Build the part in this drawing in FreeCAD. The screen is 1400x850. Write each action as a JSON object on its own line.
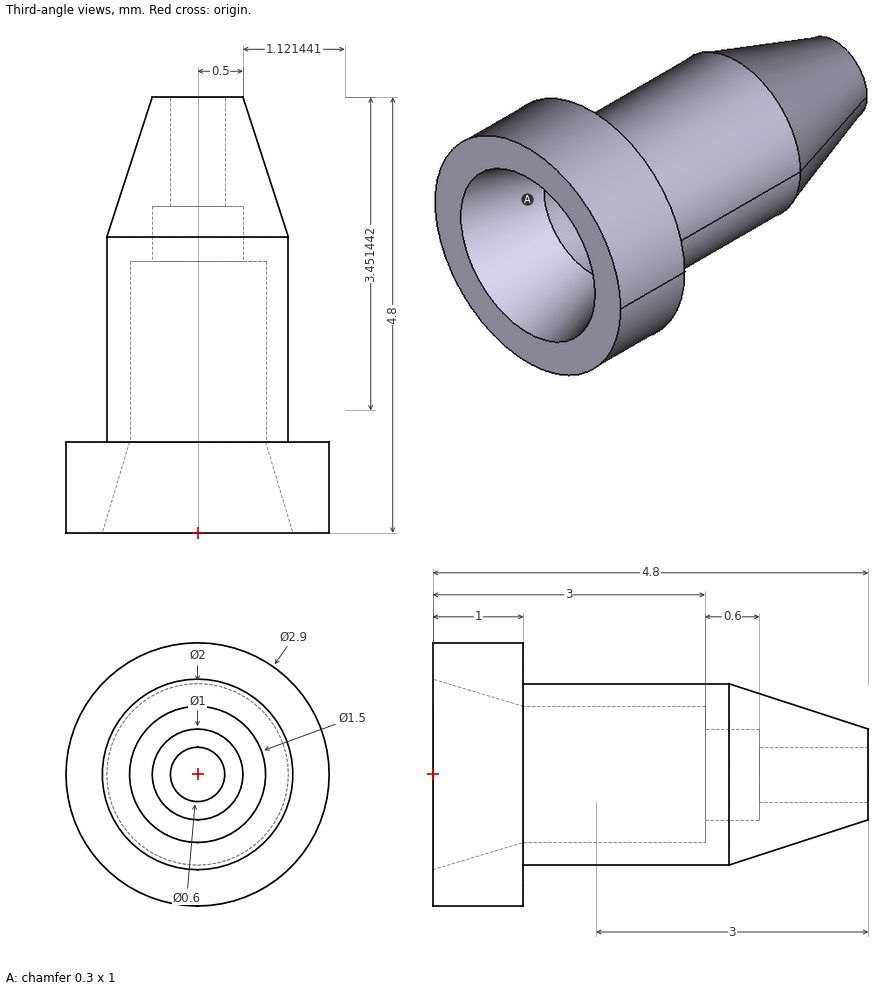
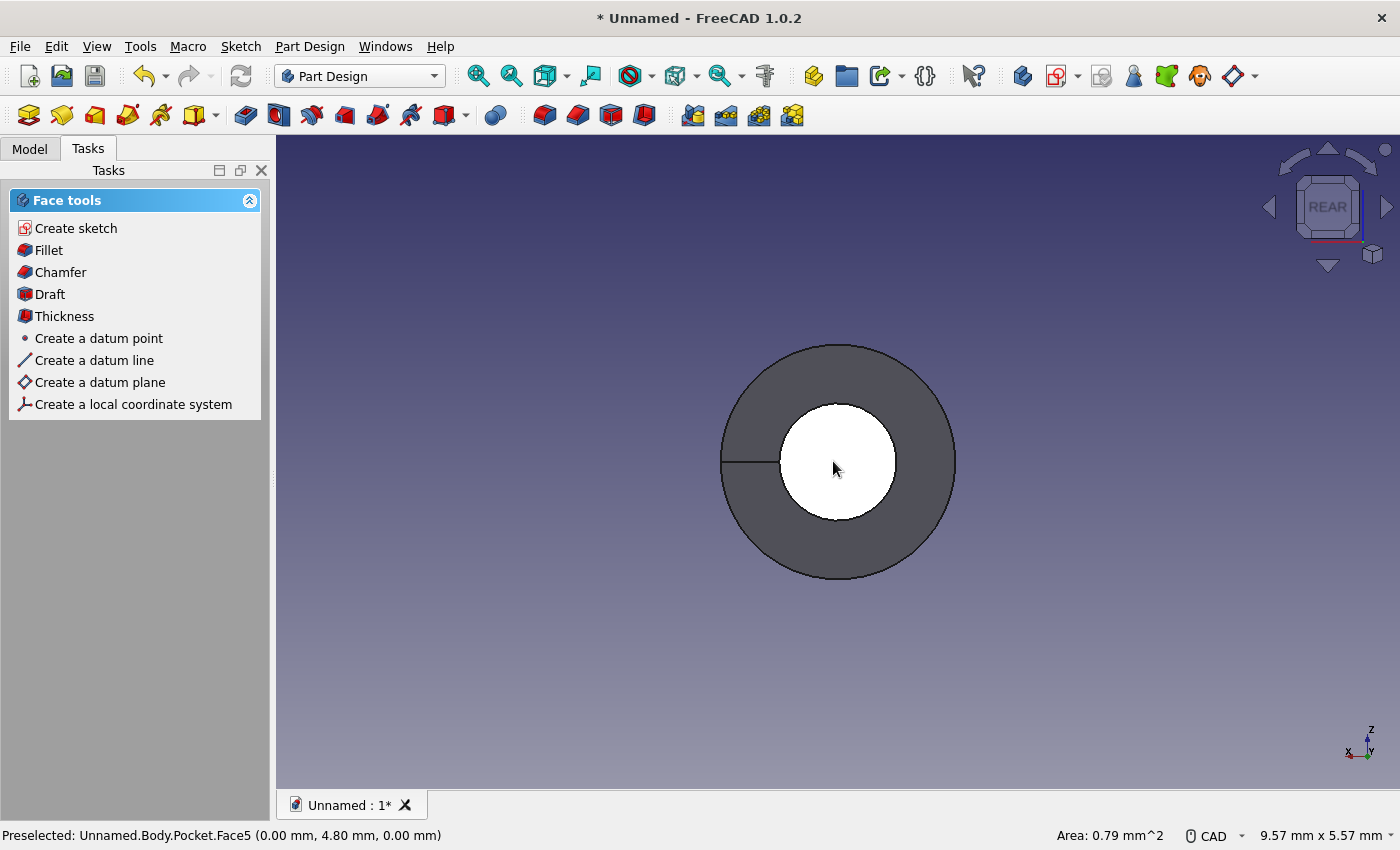
{"action": "left_click", "coordinate": [1056, 76]}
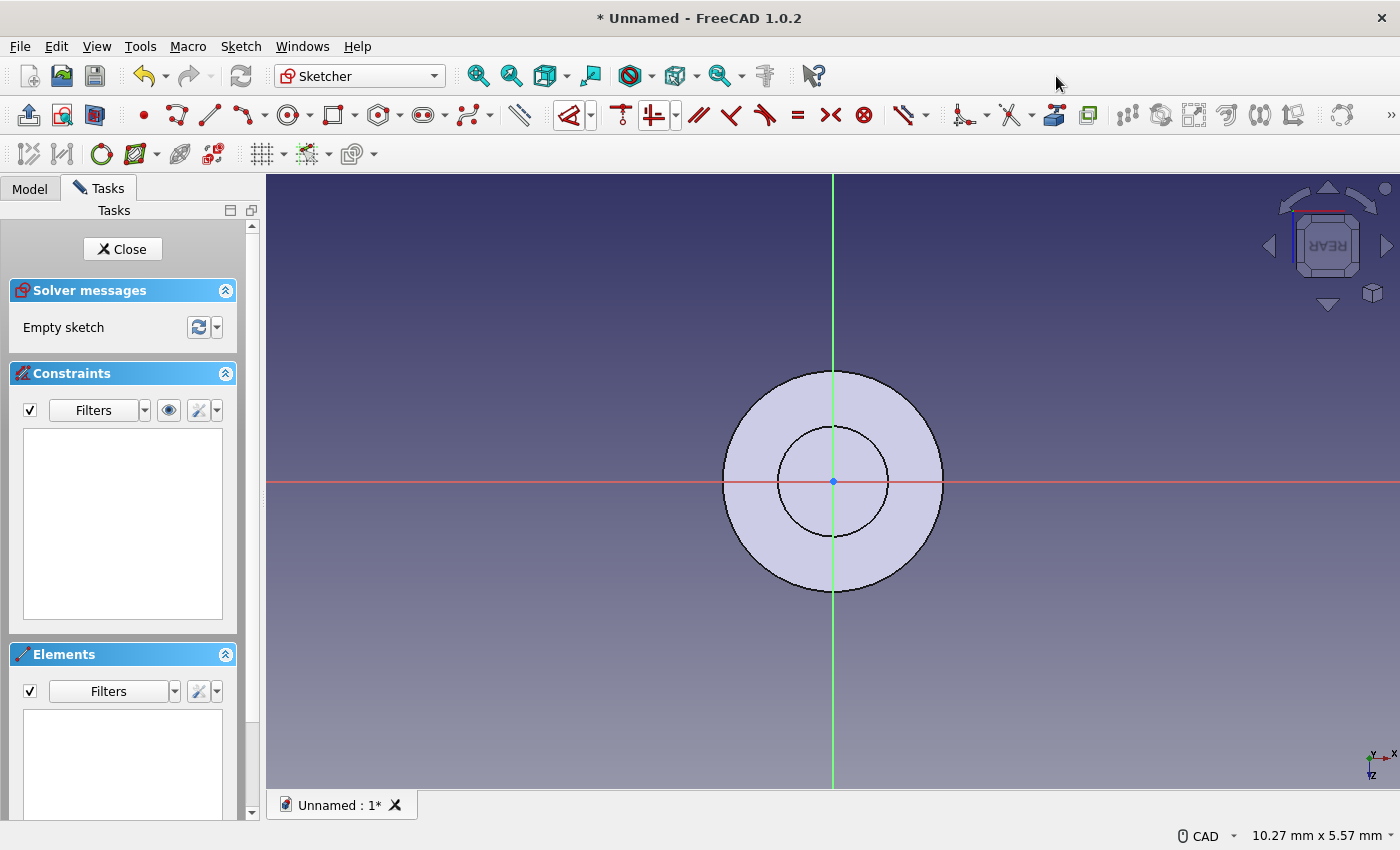
{"action": "scroll", "coordinate": [847, 481], "scroll_direction": "up", "scroll_amount": 9}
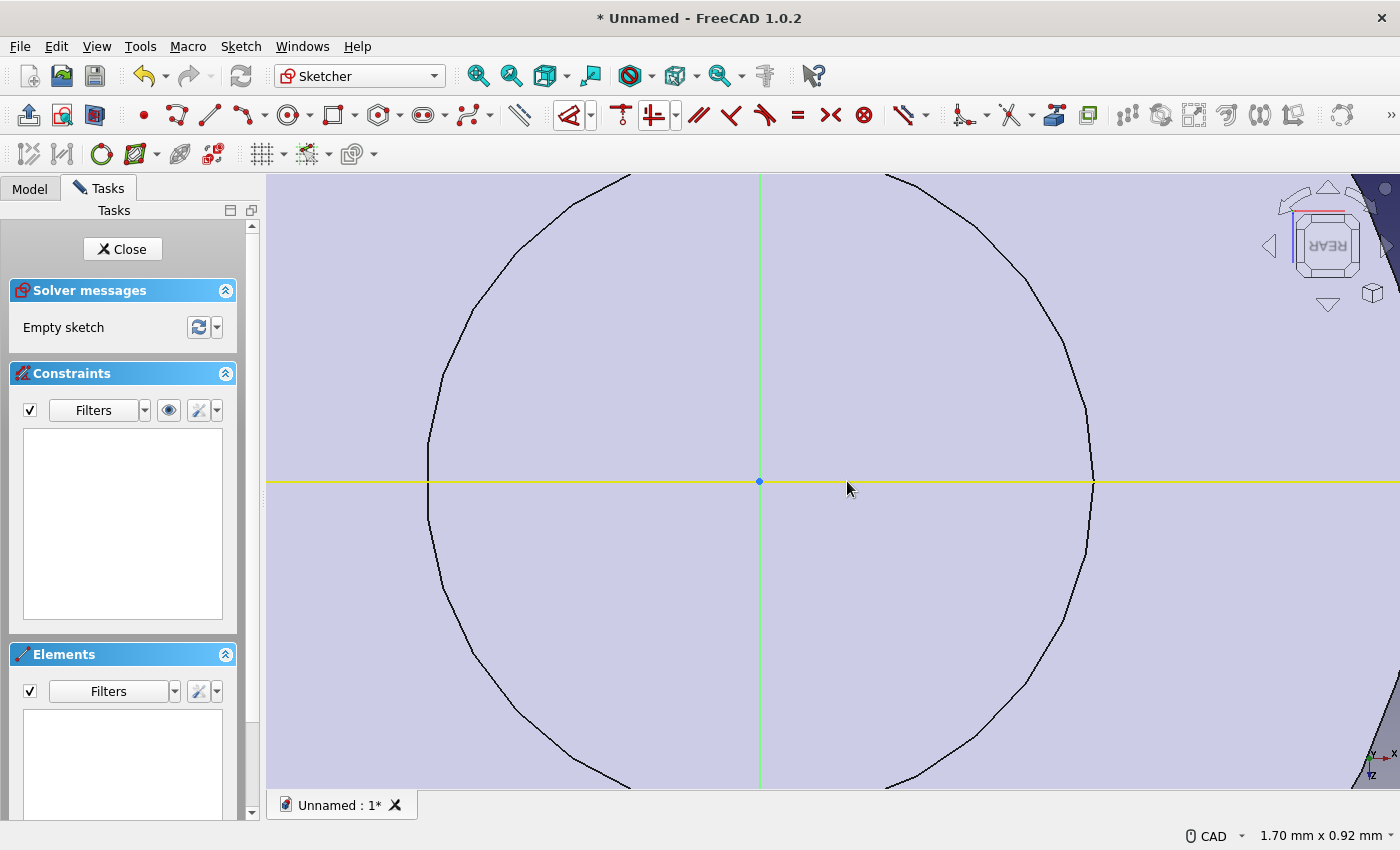
{"action": "left_click", "coordinate": [288, 116]}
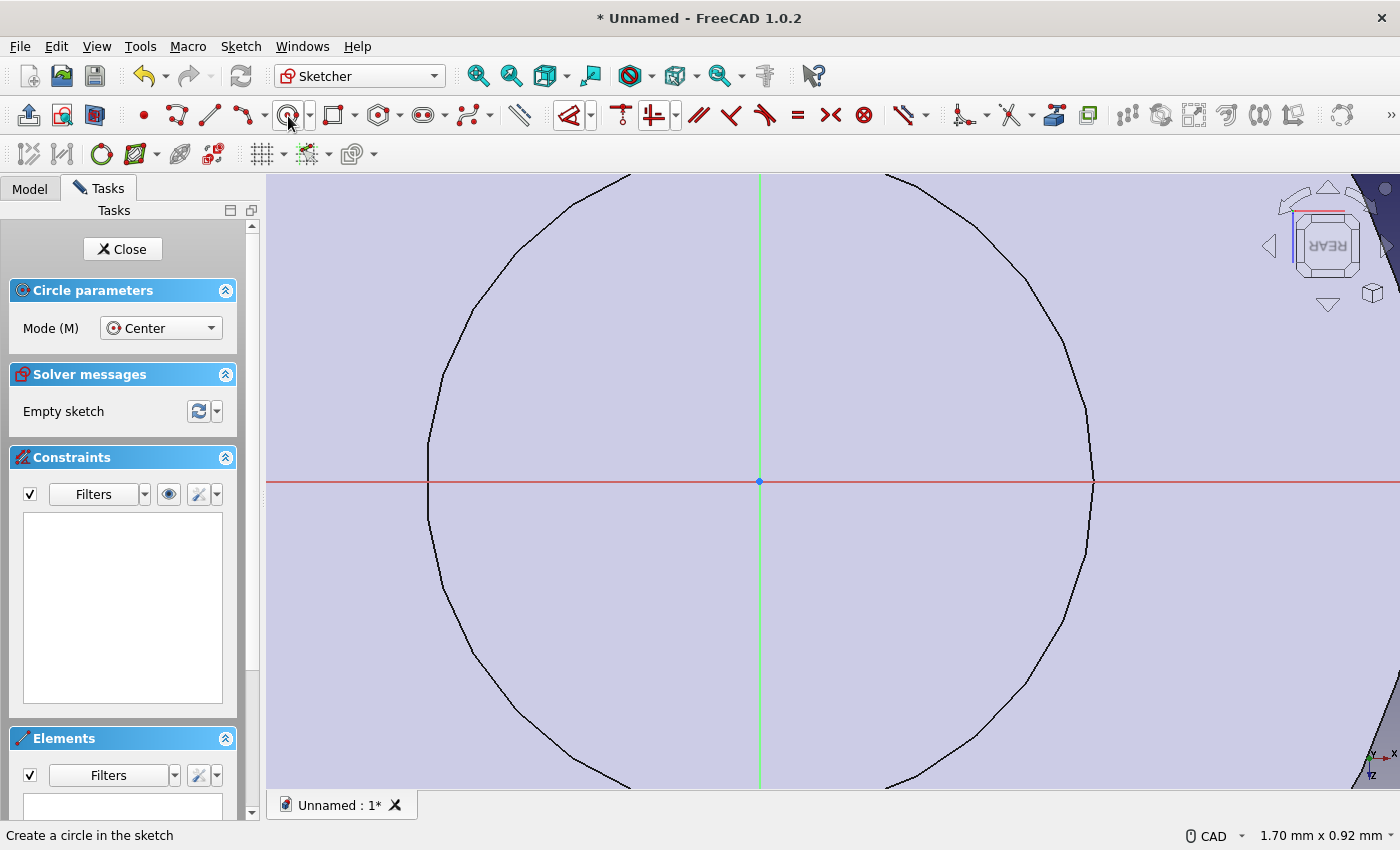
{"action": "left_click", "coordinate": [760, 481]}
{"action": "left_click", "coordinate": [901, 340]}
{"action": "key", "text": "Escape"}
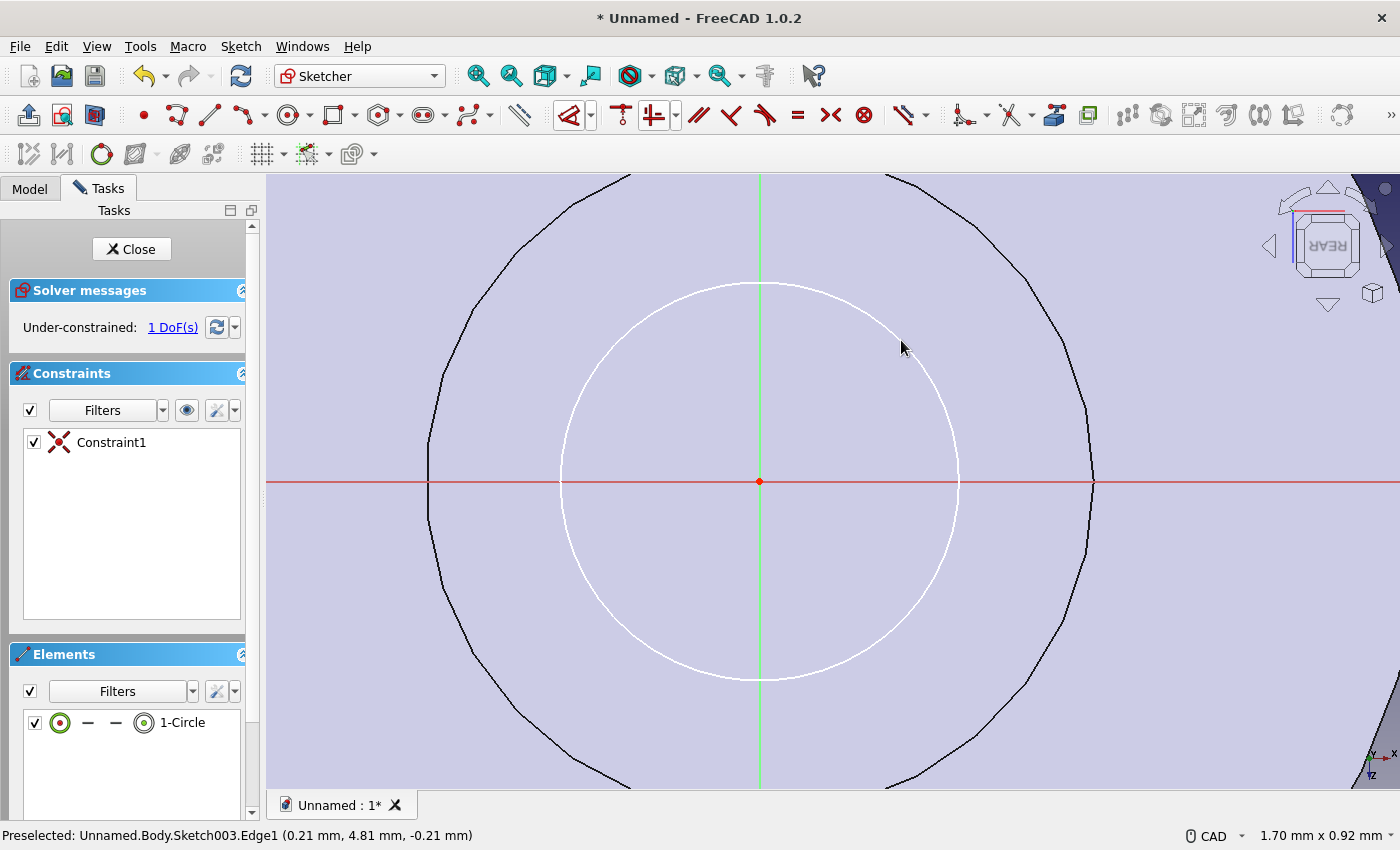
{"action": "left_click", "coordinate": [900, 340]}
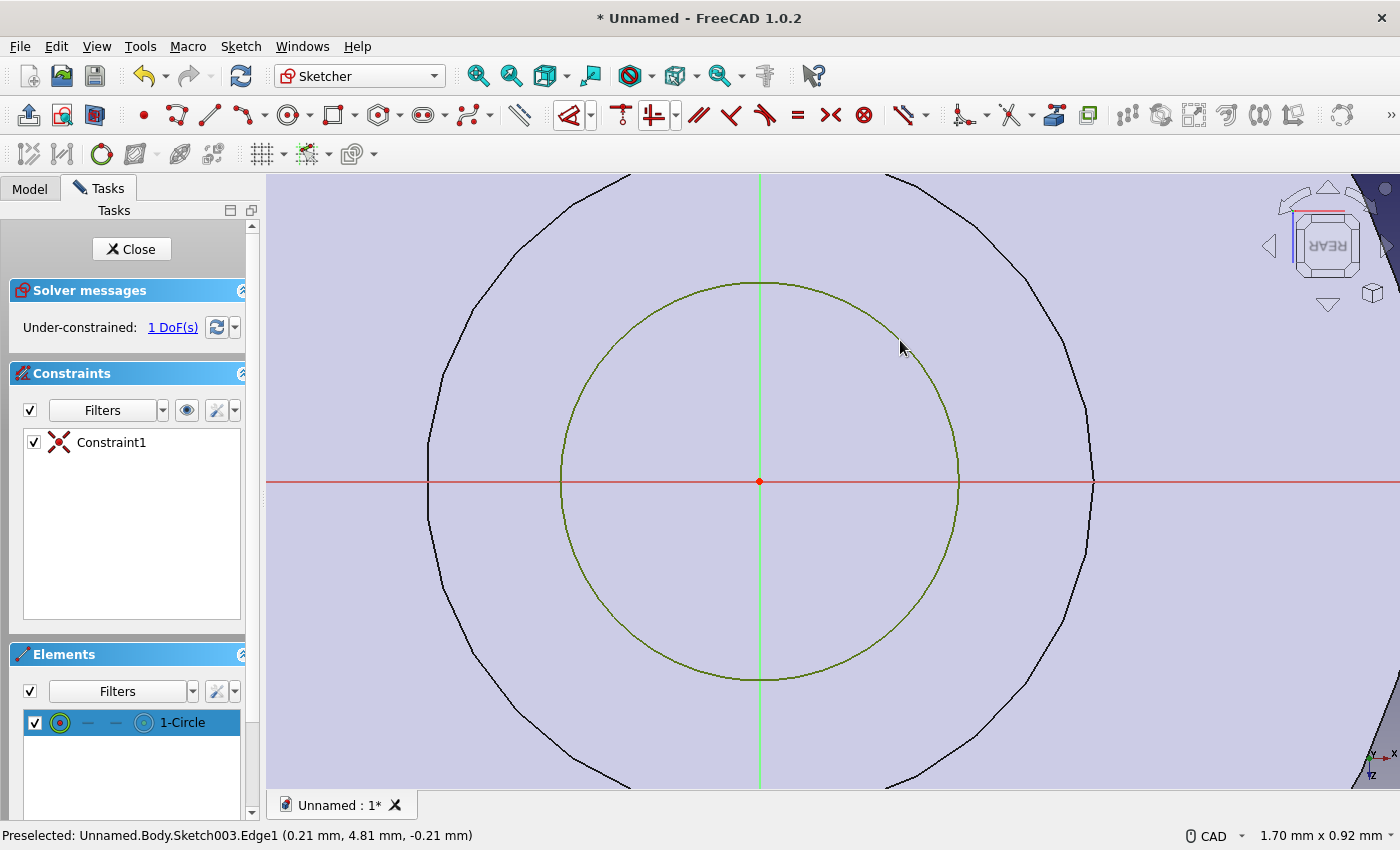
{"action": "left_click", "coordinate": [590, 116]}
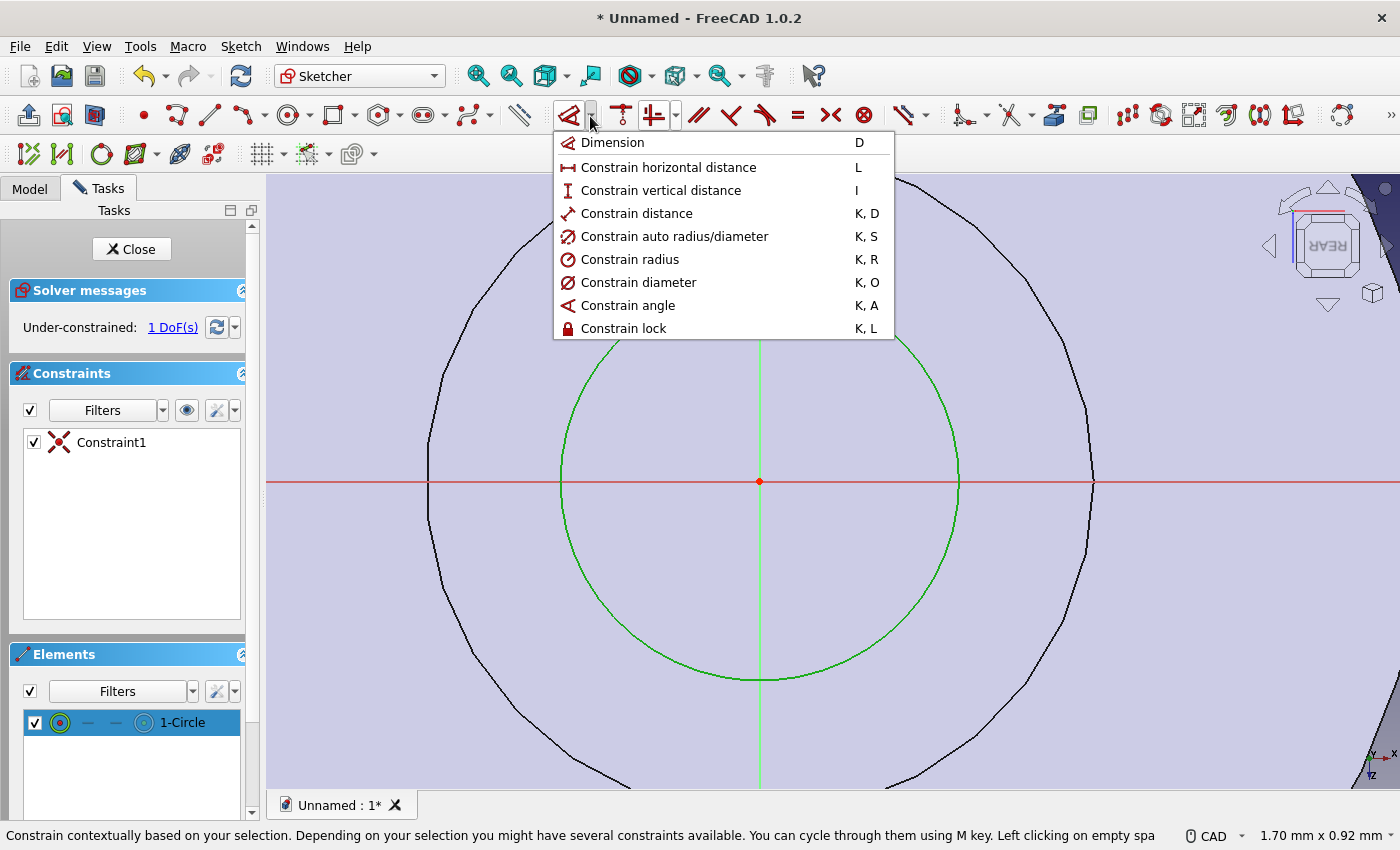
{"action": "left_click", "coordinate": [724, 282]}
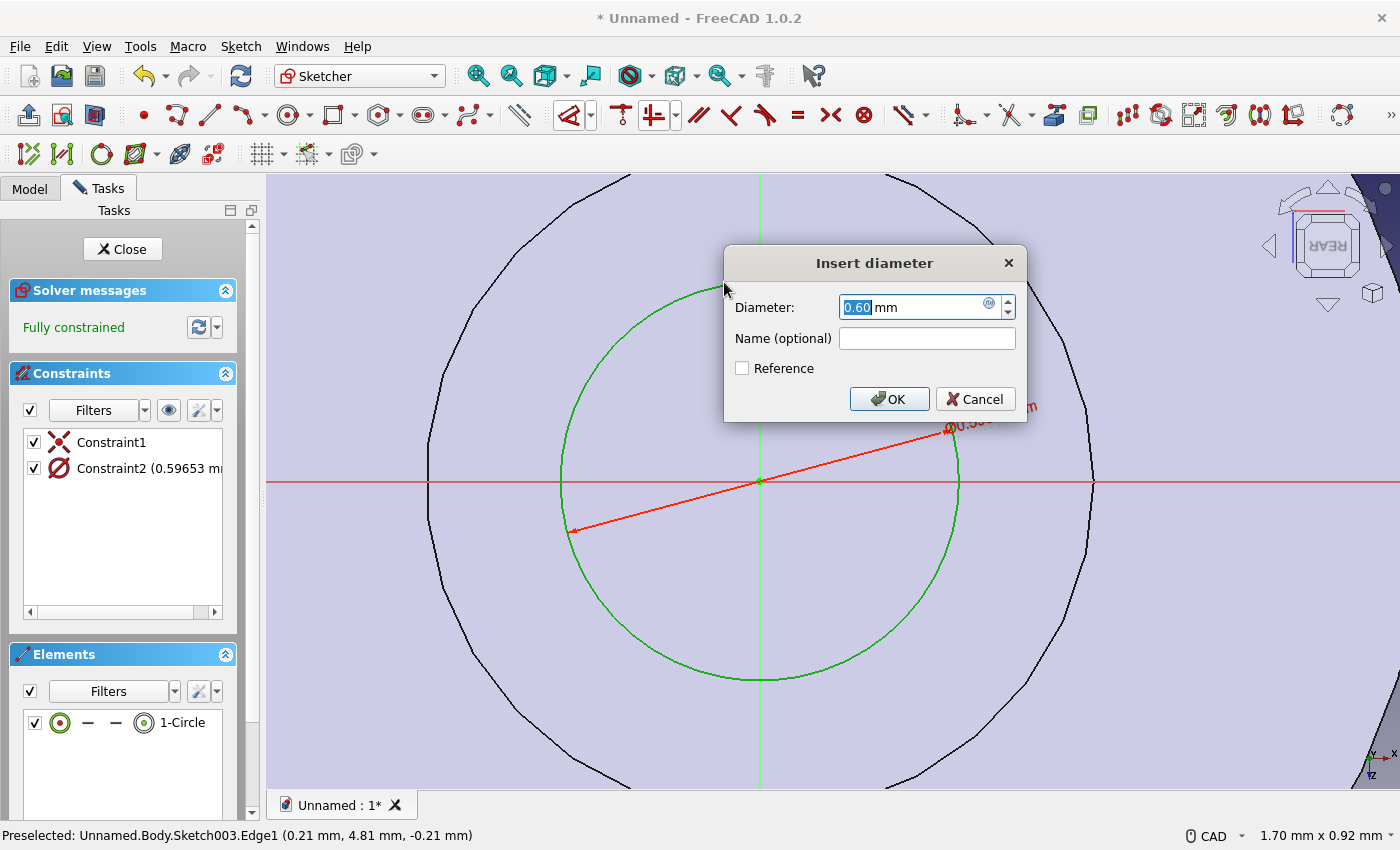
{"action": "type", "text": "0.6"}
{"action": "key", "text": "Return"}